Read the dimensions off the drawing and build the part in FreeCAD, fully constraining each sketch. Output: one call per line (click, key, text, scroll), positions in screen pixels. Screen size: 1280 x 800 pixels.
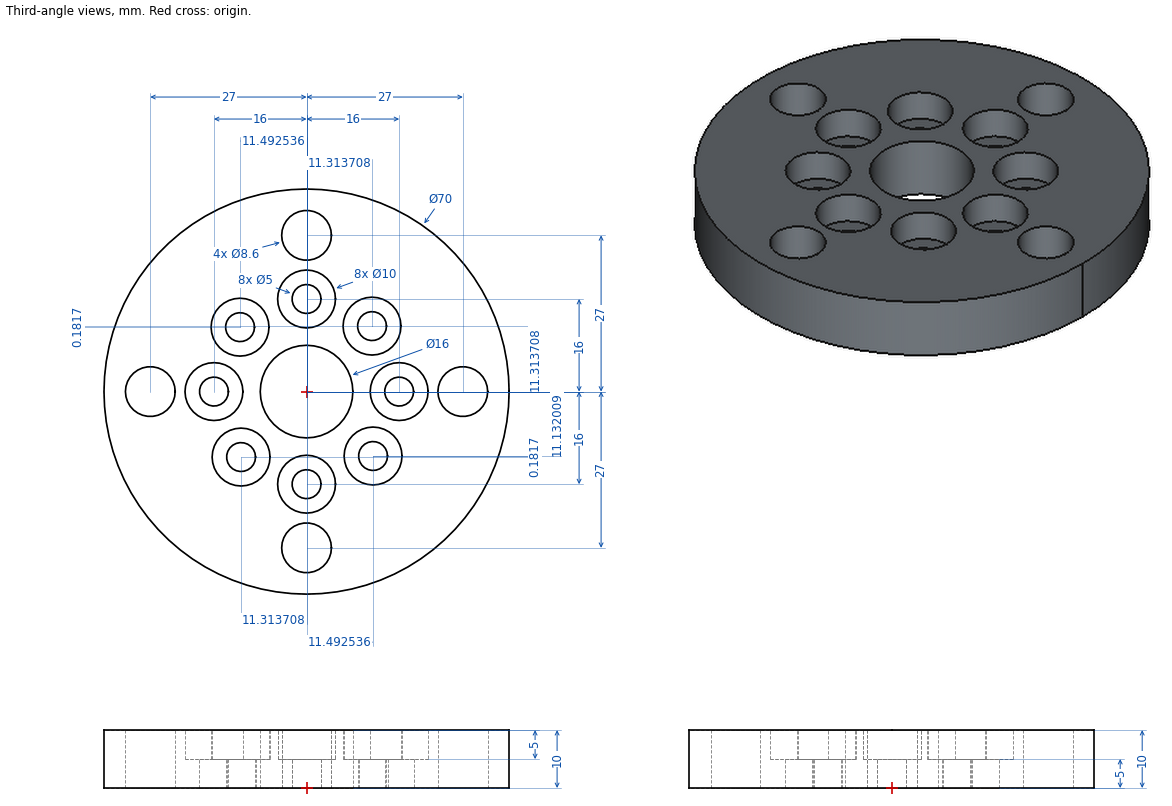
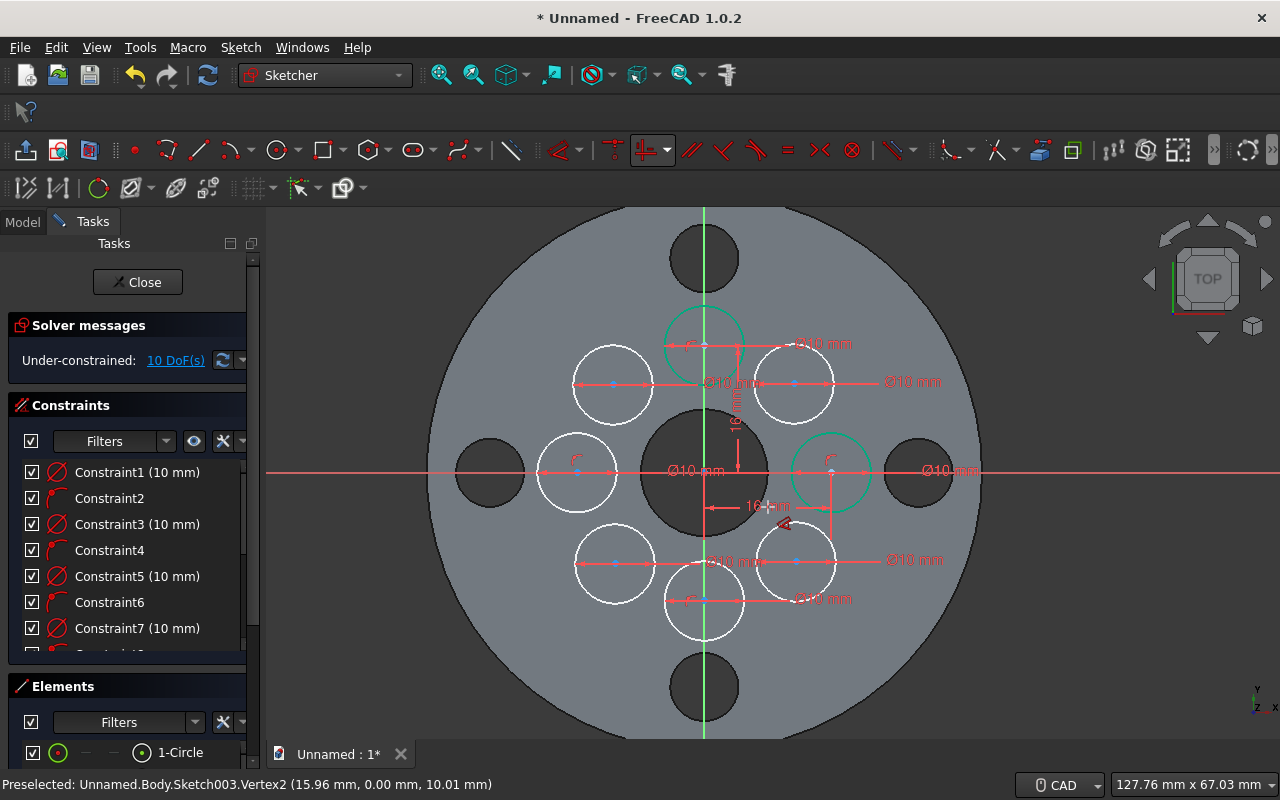
click(704, 601)
click(738, 537)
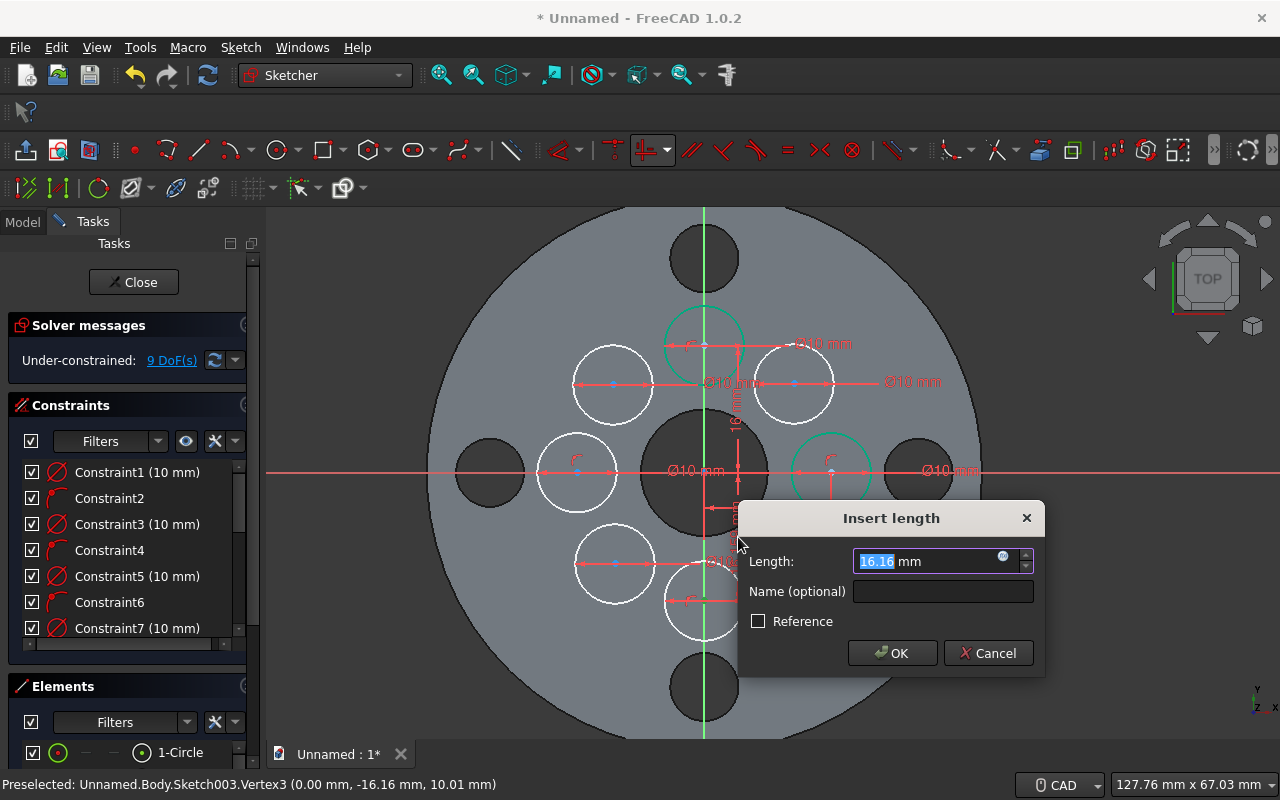
text(16)
key(Return)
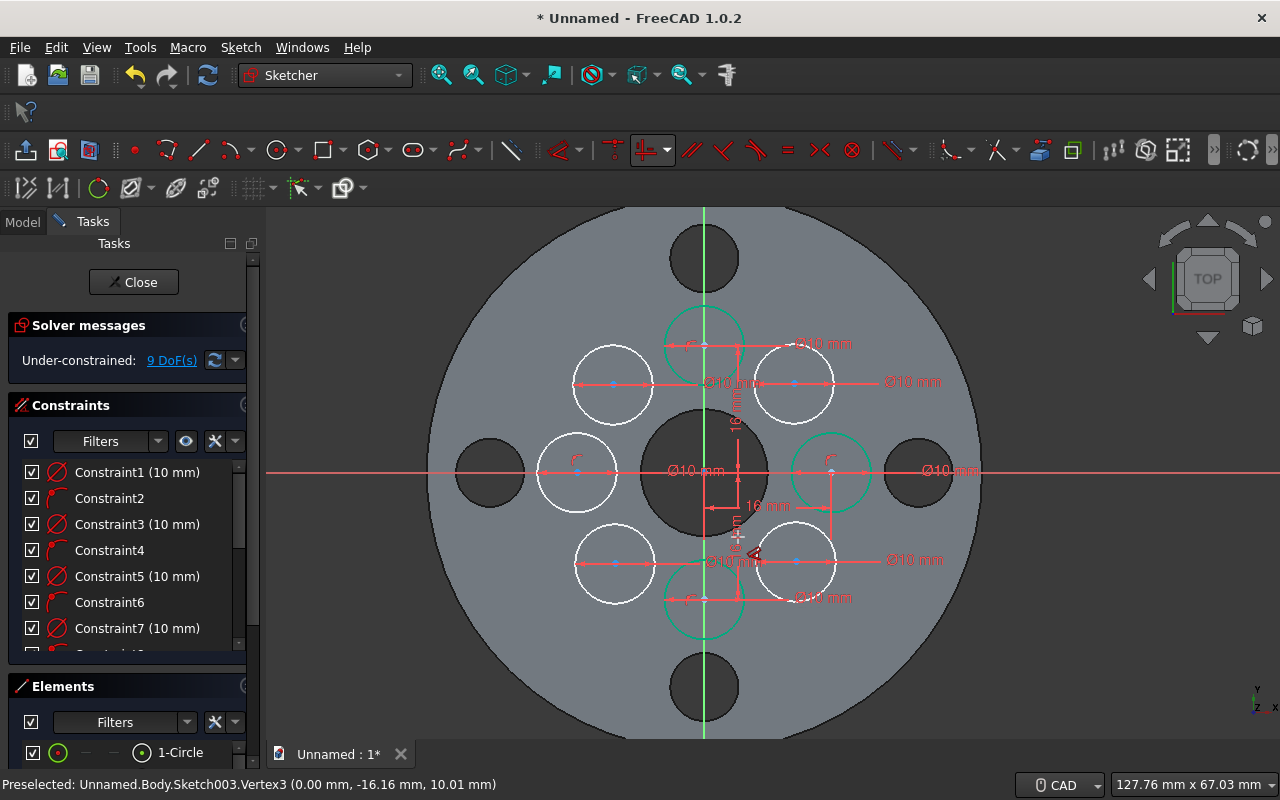
click(577, 473)
click(641, 507)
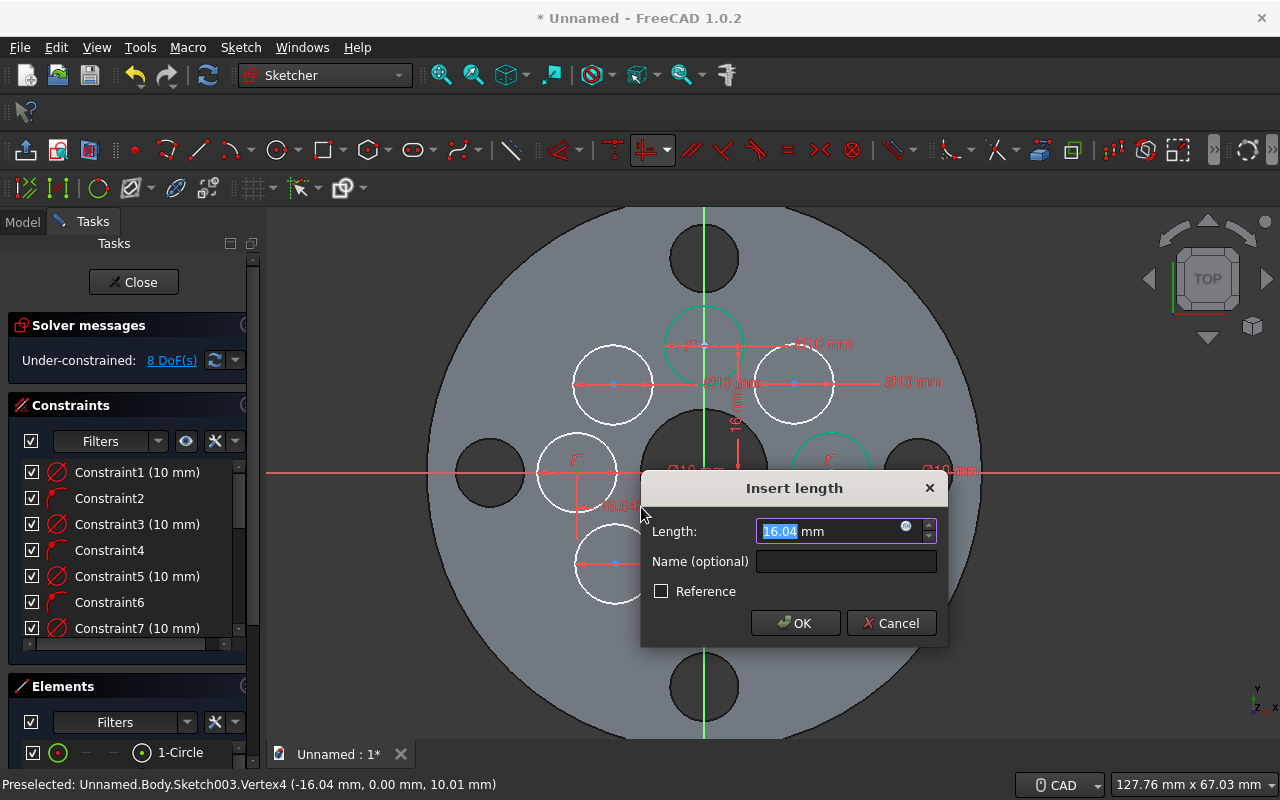
text(16)
key(Return)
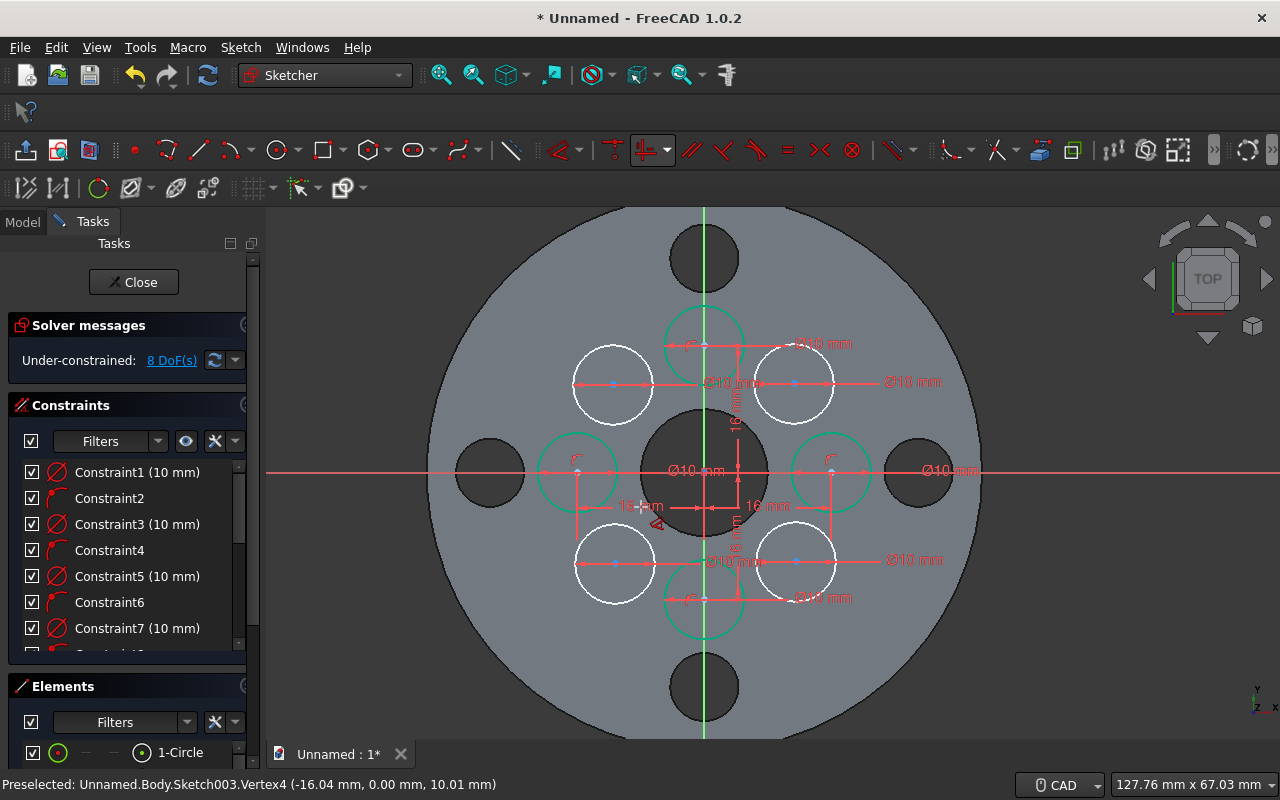
scroll(794, 384, up, 17)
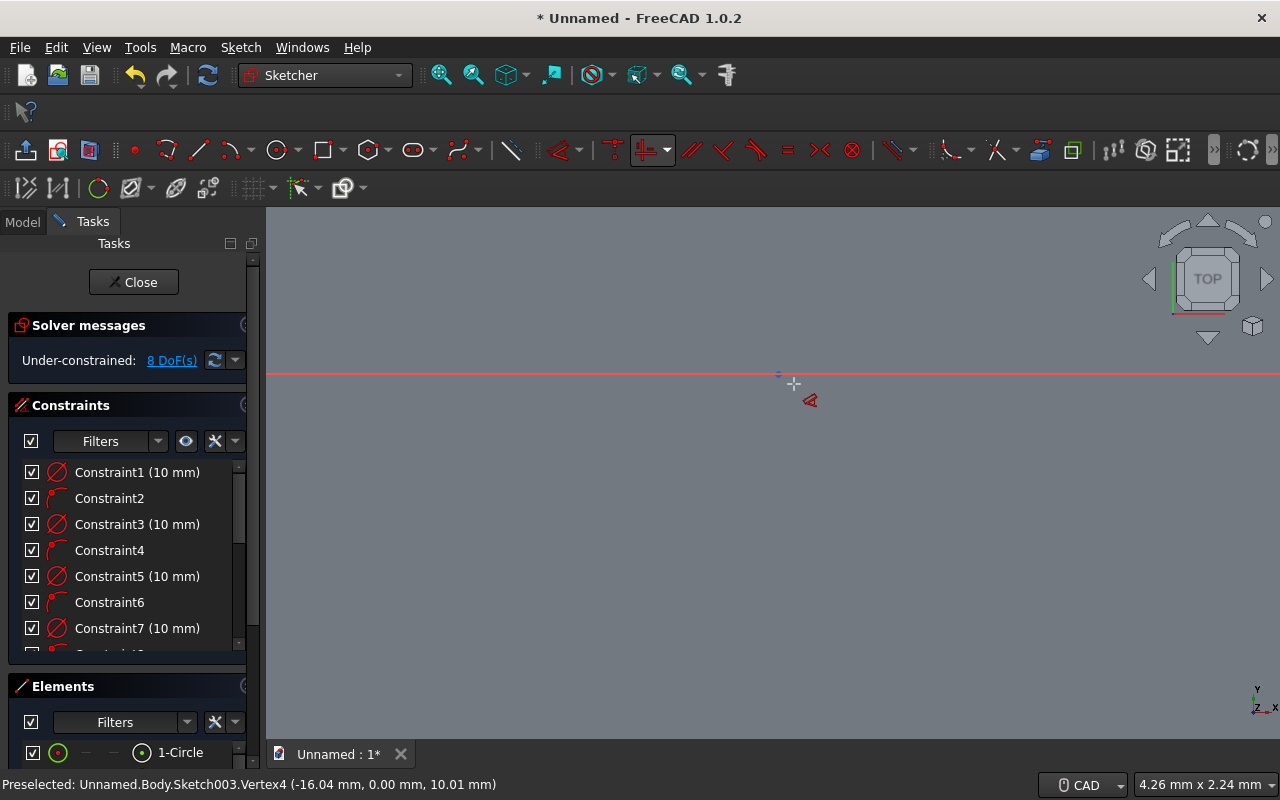
click(779, 374)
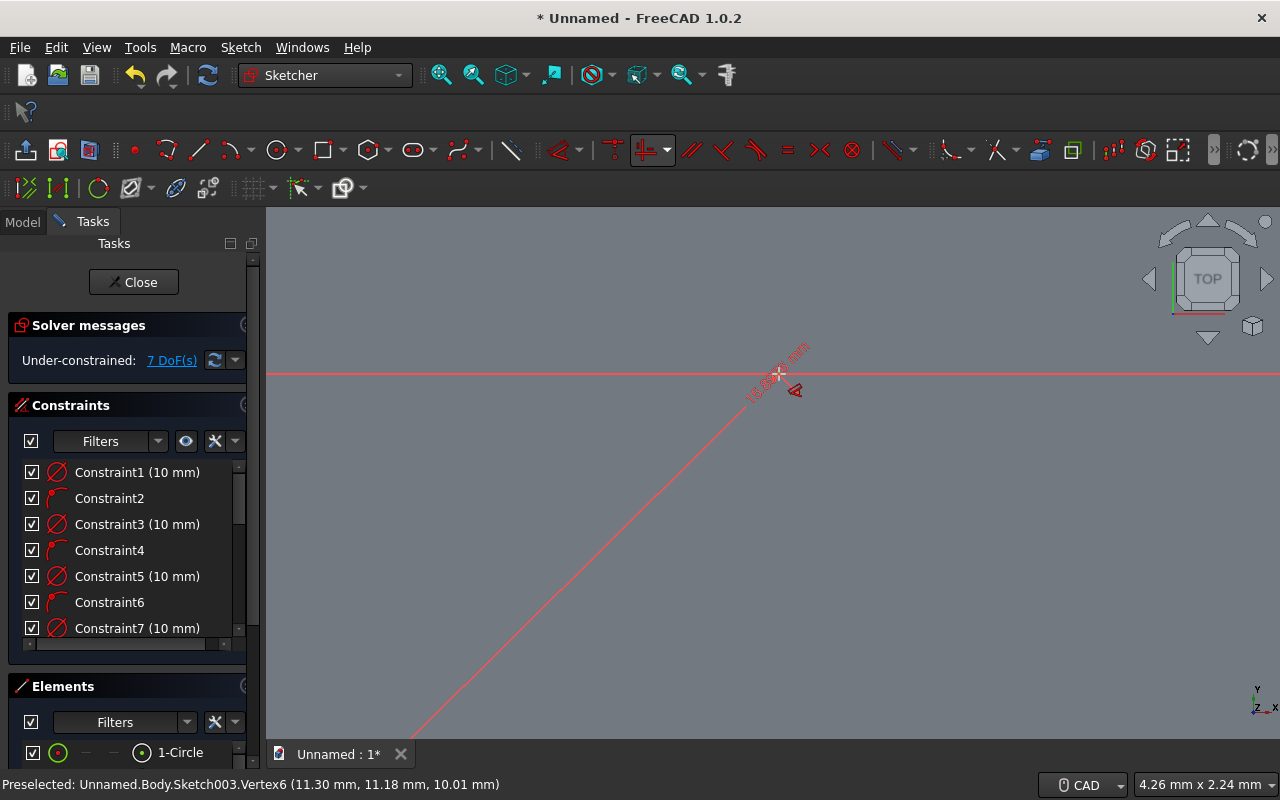
scroll(816, 364, down, 16)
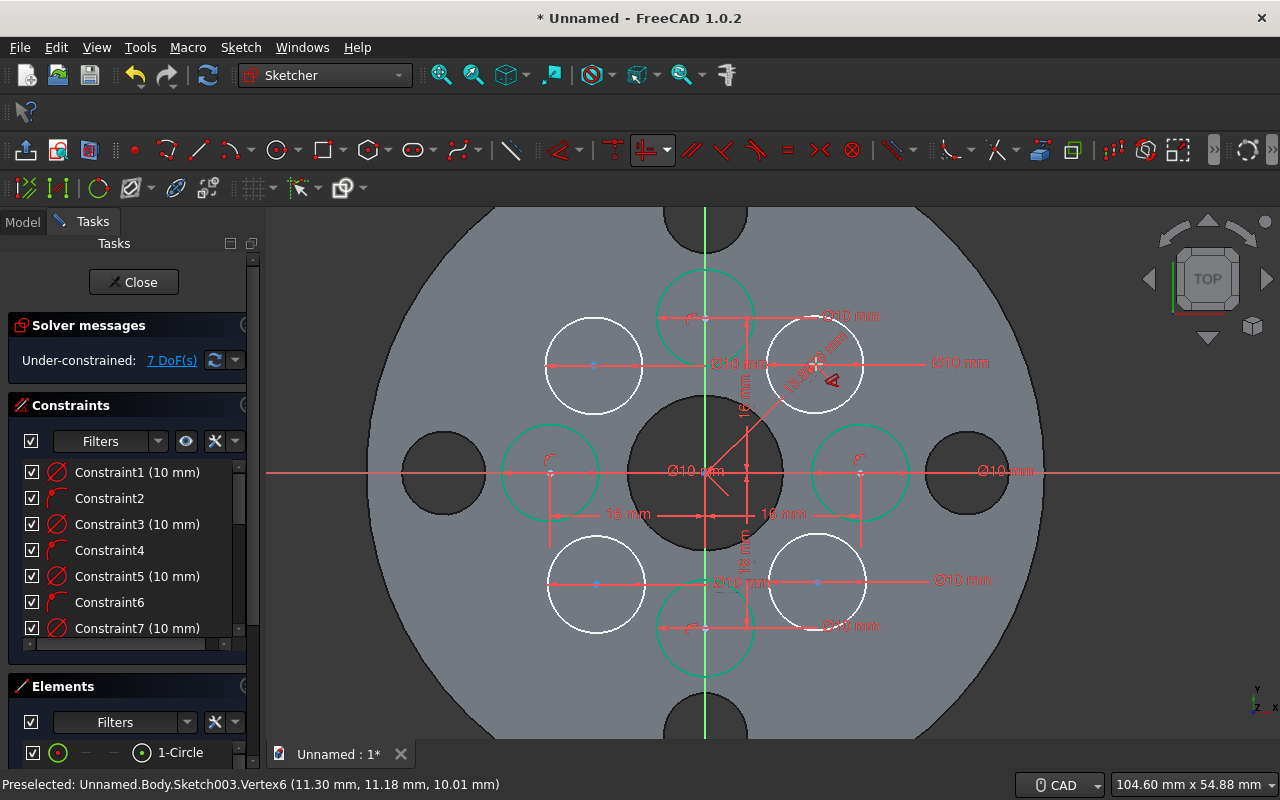
scroll(594, 366, up, 16)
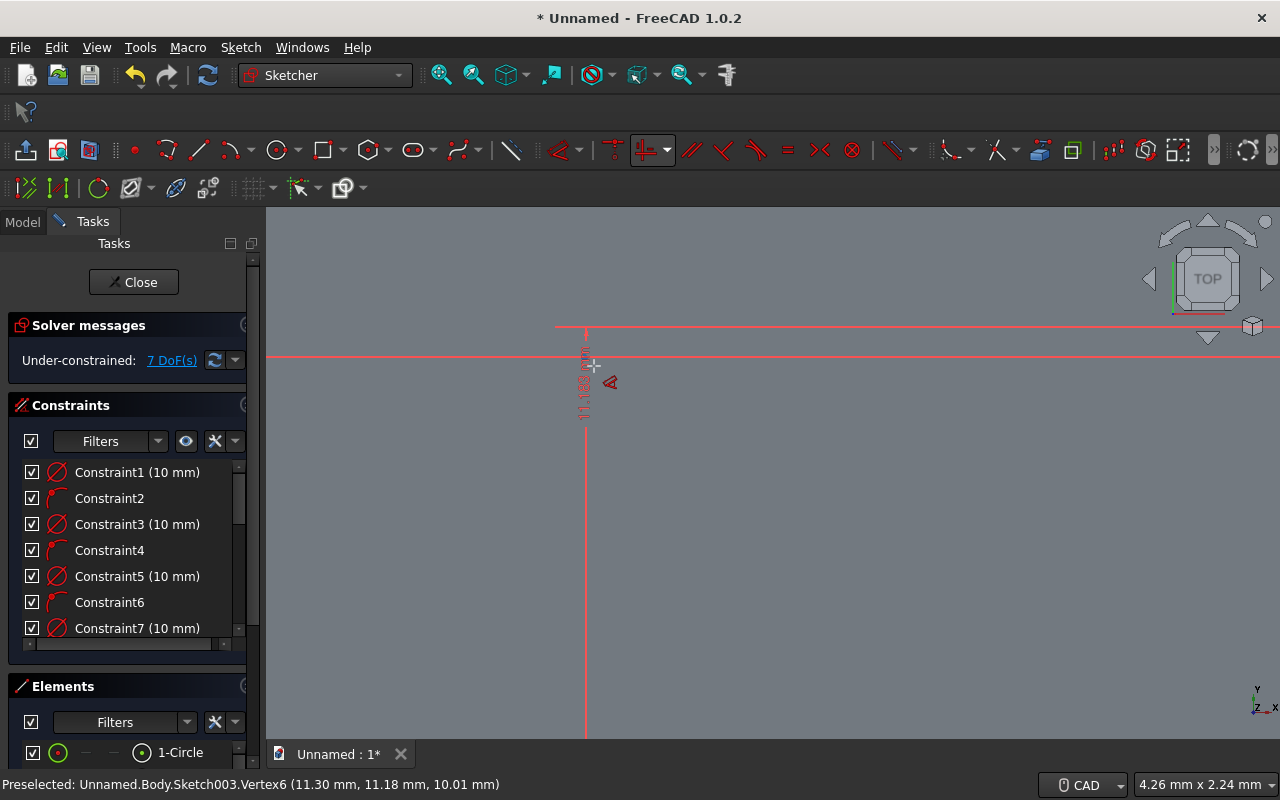
click(585, 357)
click(551, 342)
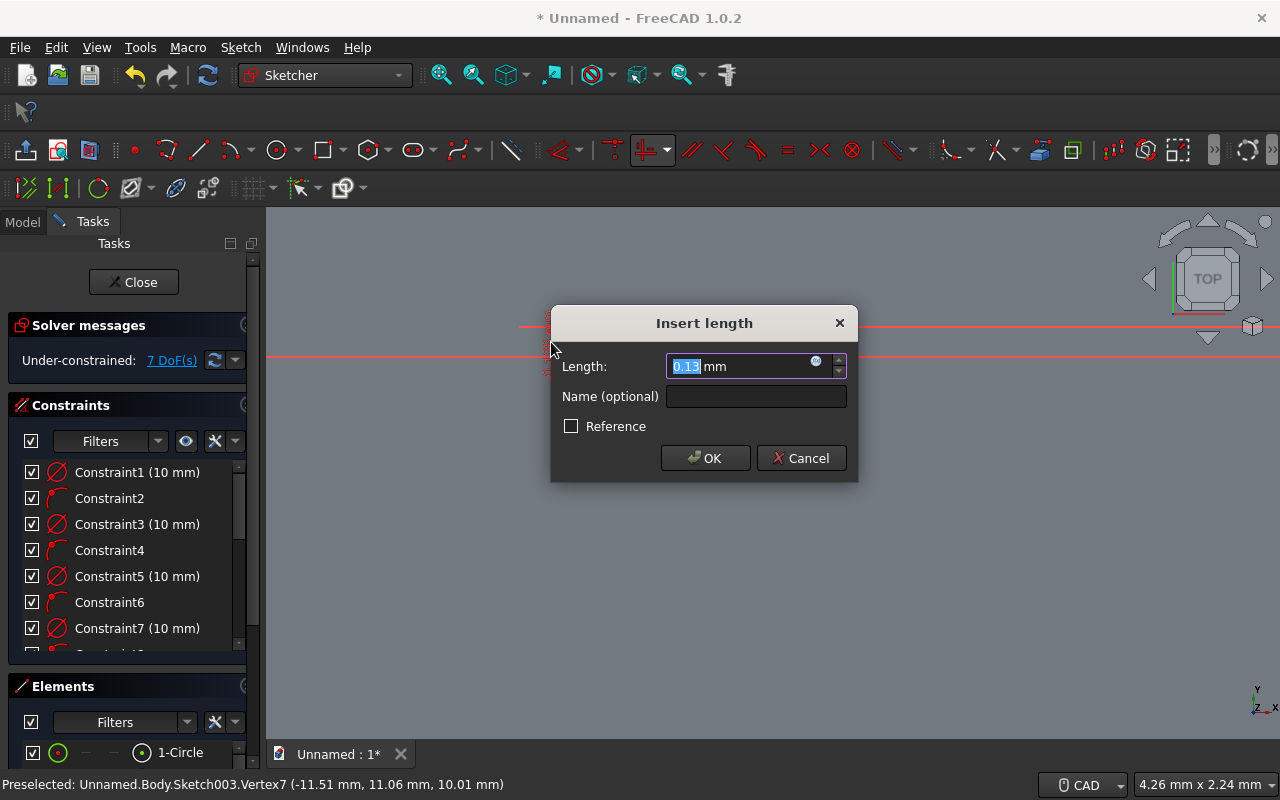
text(0.1817)
key(Return)